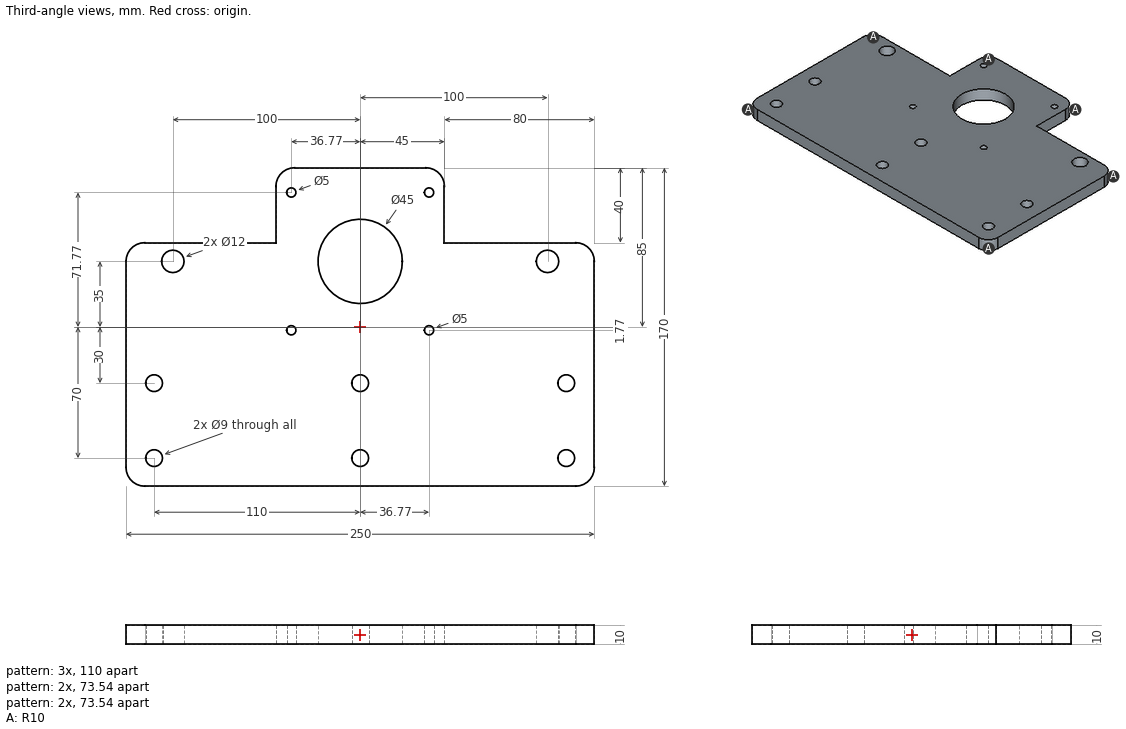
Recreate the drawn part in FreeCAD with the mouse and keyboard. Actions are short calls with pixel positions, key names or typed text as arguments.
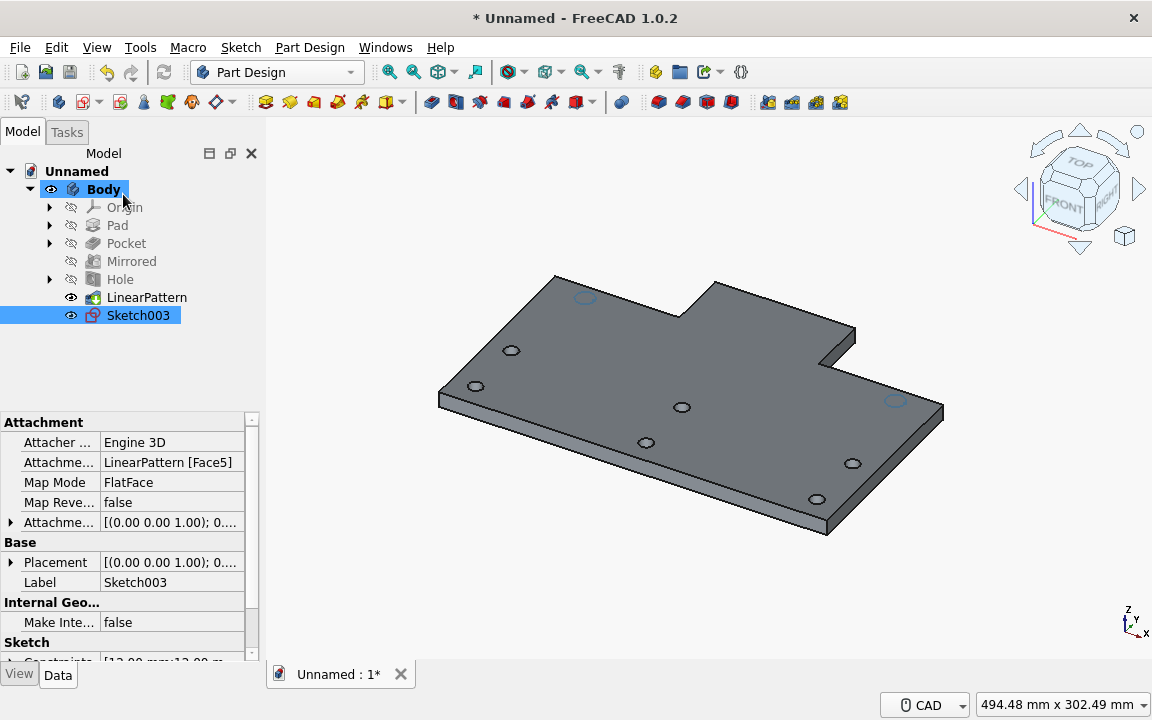
click(432, 102)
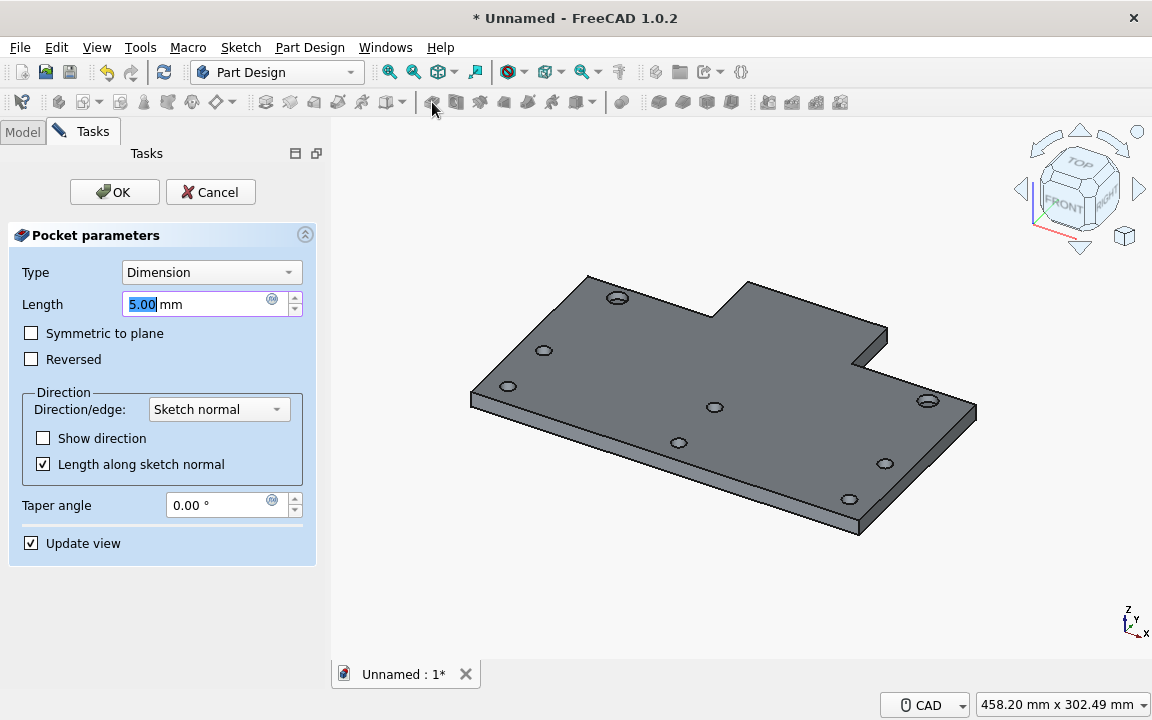
click(212, 272)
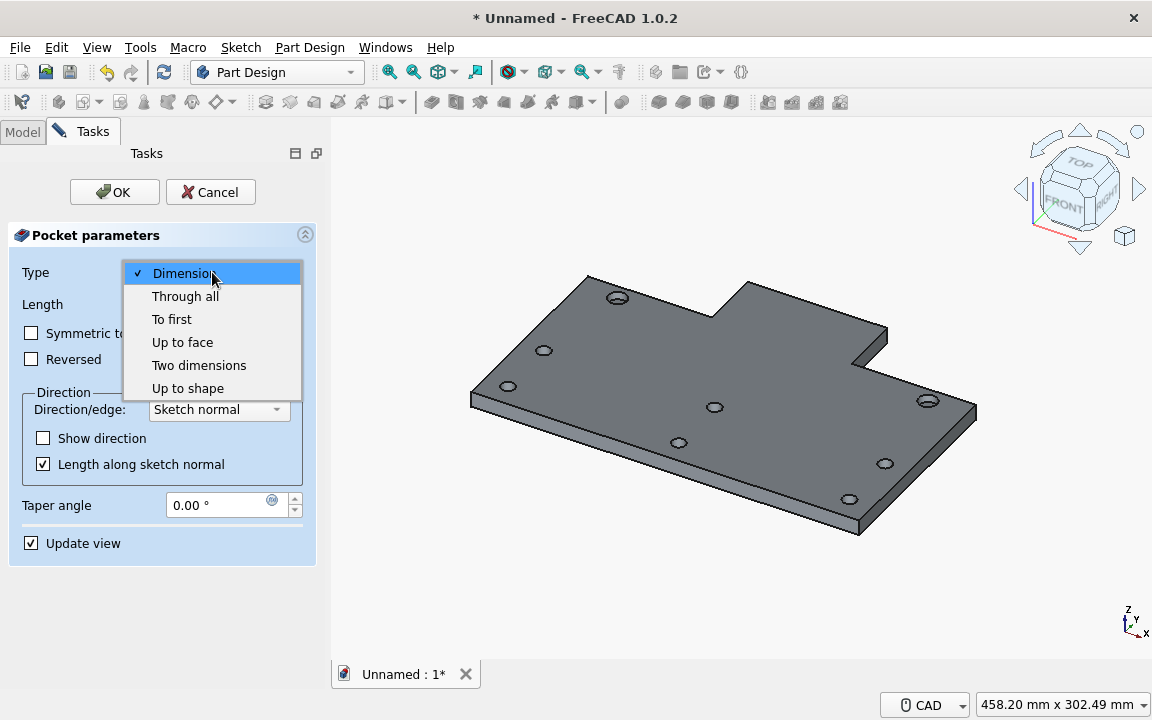
click(212, 296)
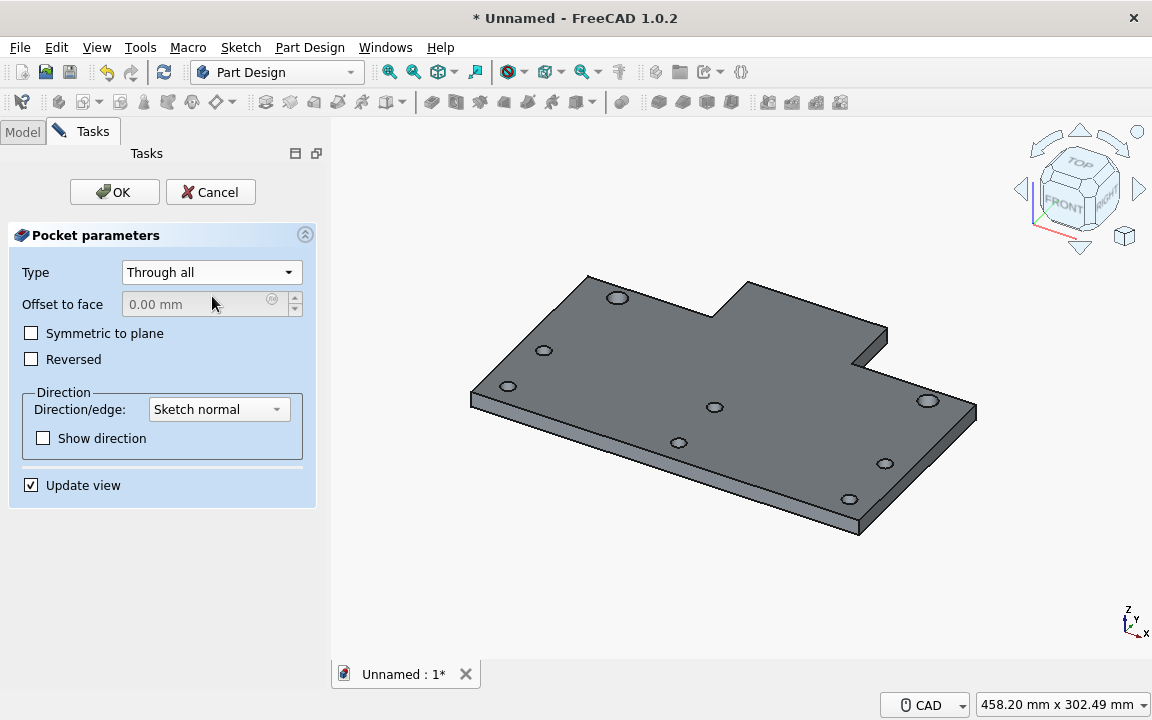
click(115, 192)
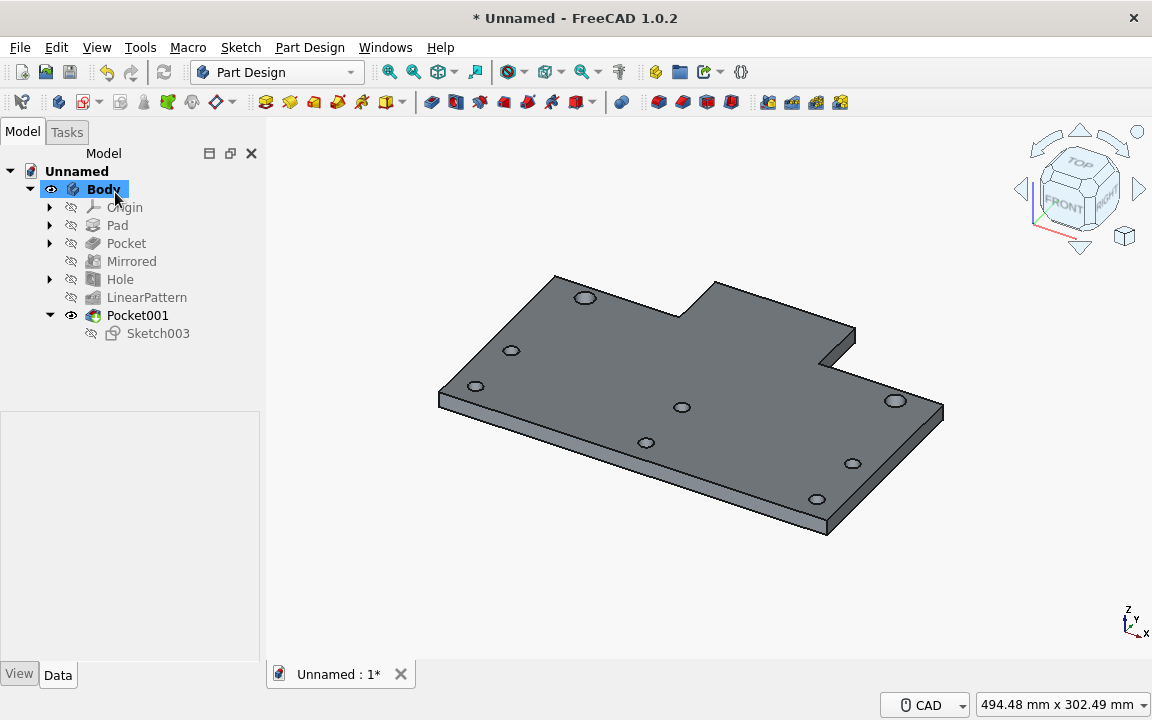
click(731, 358)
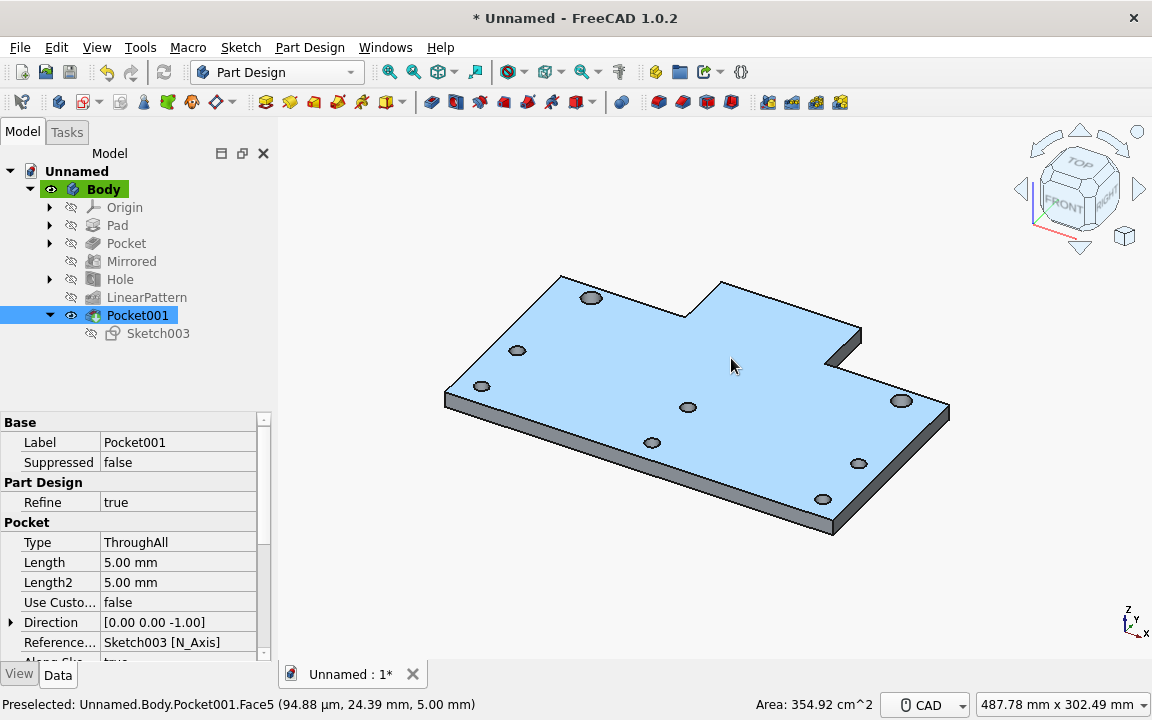
click(84, 102)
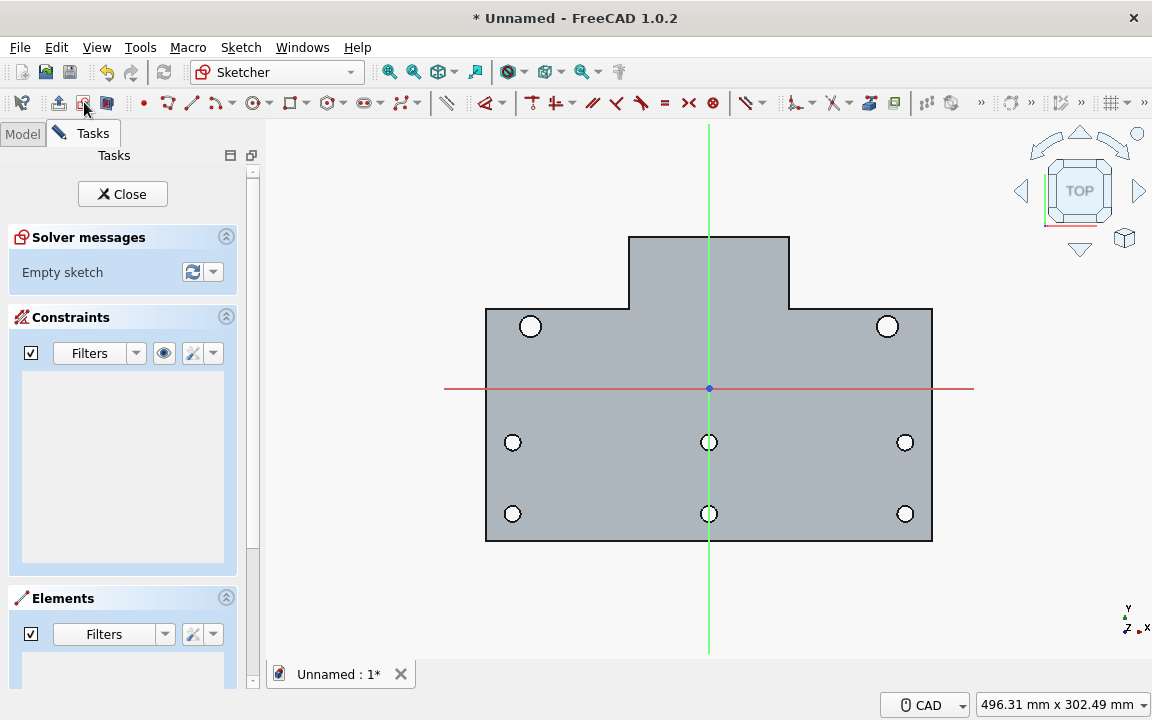
scroll(739, 316, up, 6)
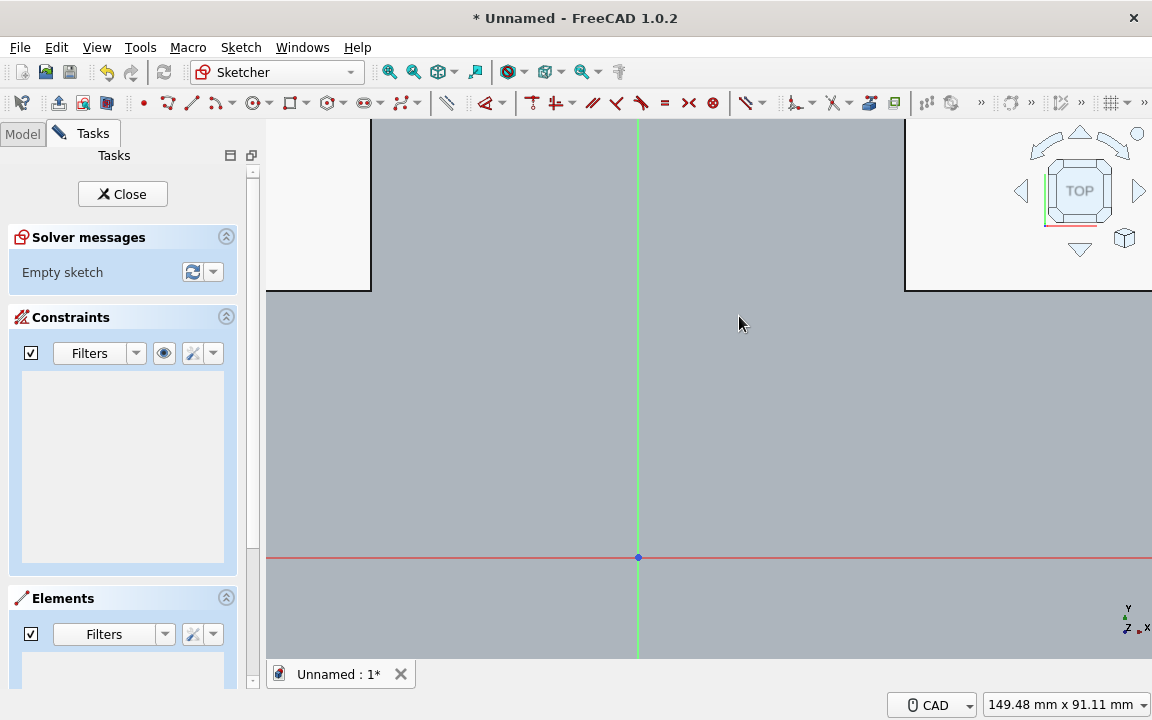
click(254, 104)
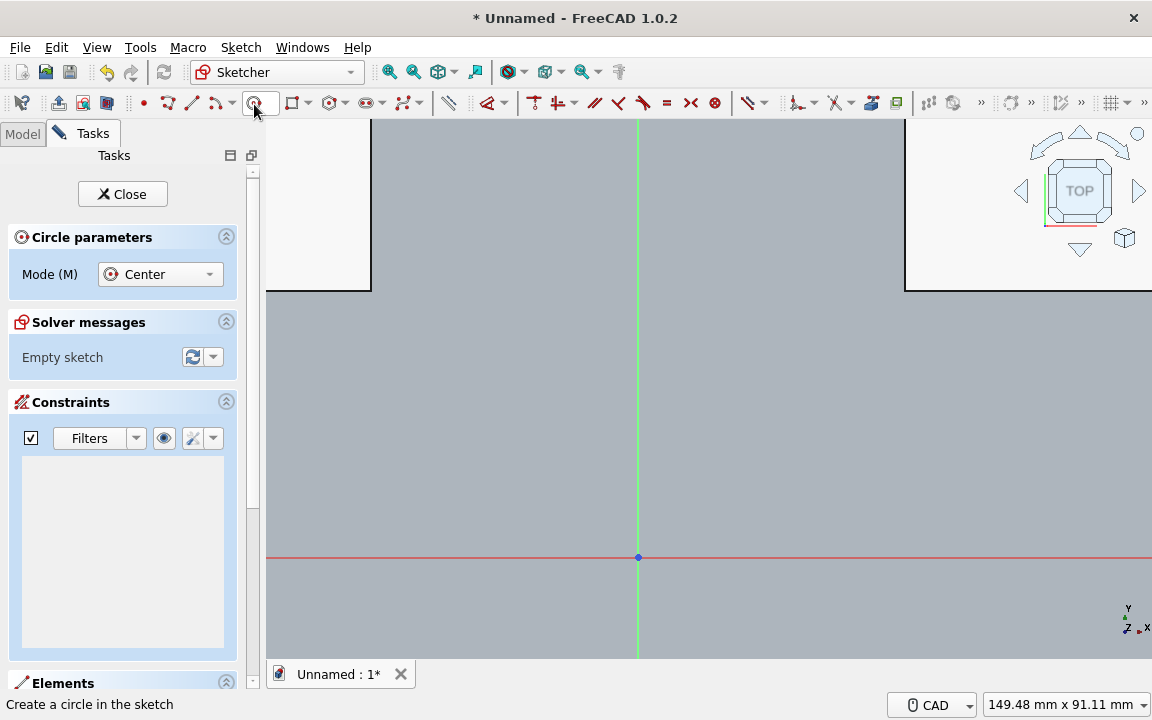
click(638, 350)
move(732, 256)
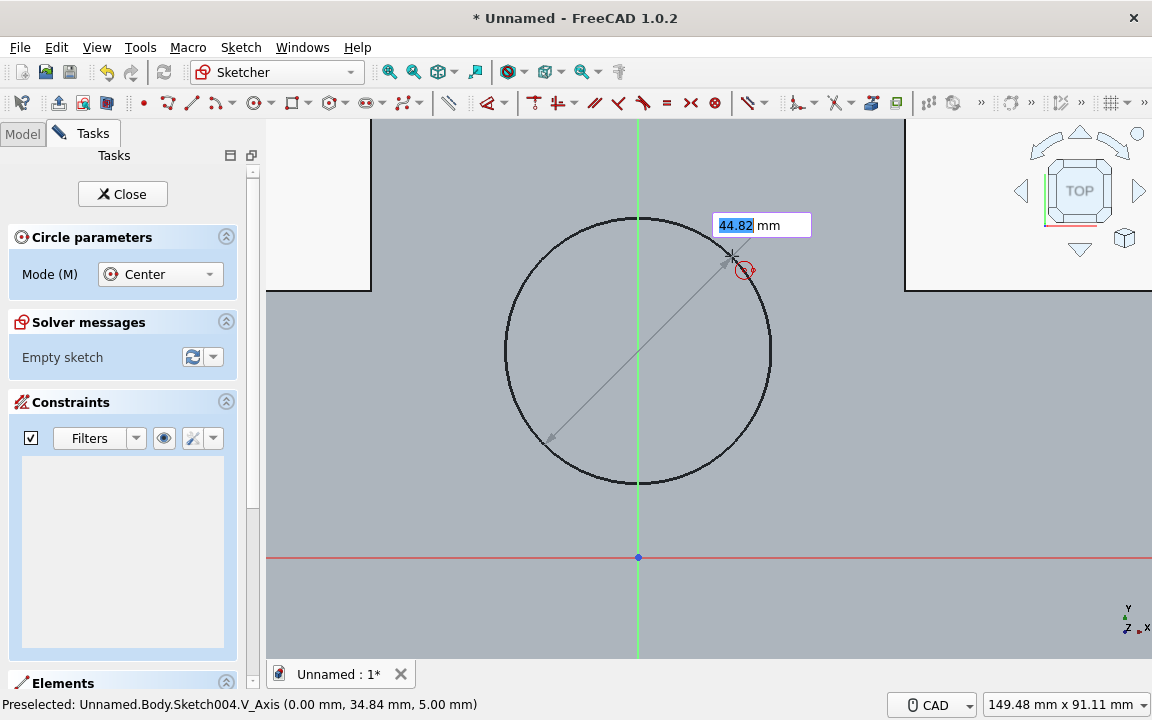
text(45)
key(Return)
key(Escape)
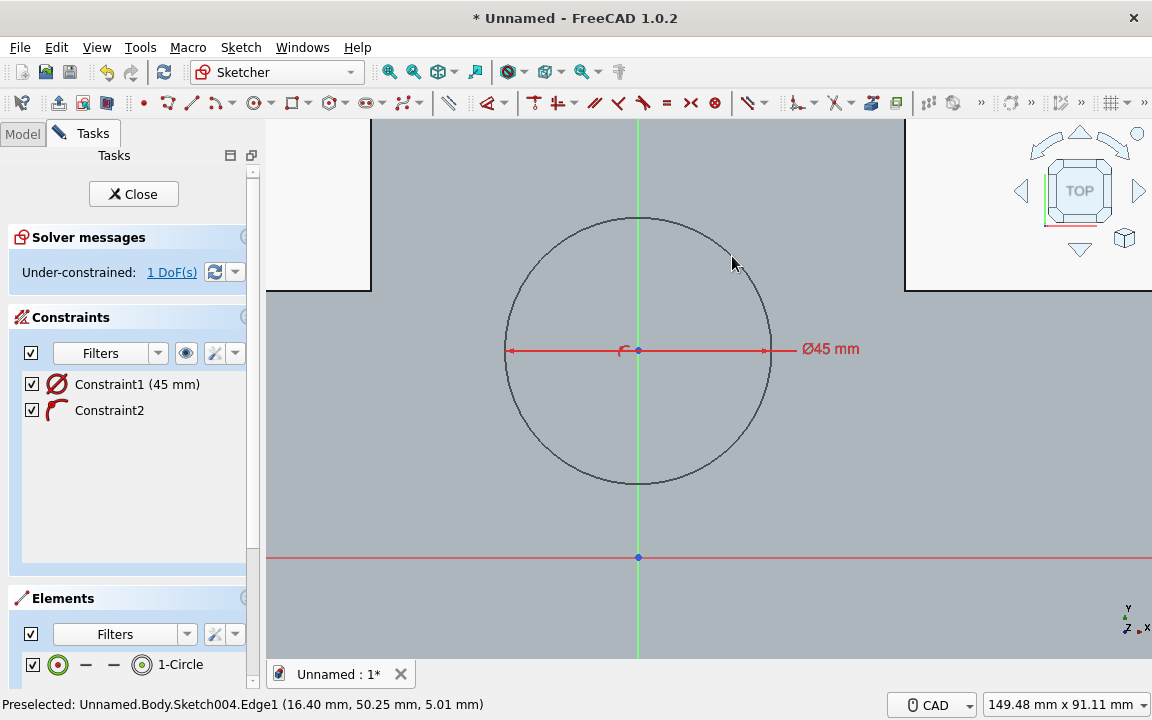
click(488, 104)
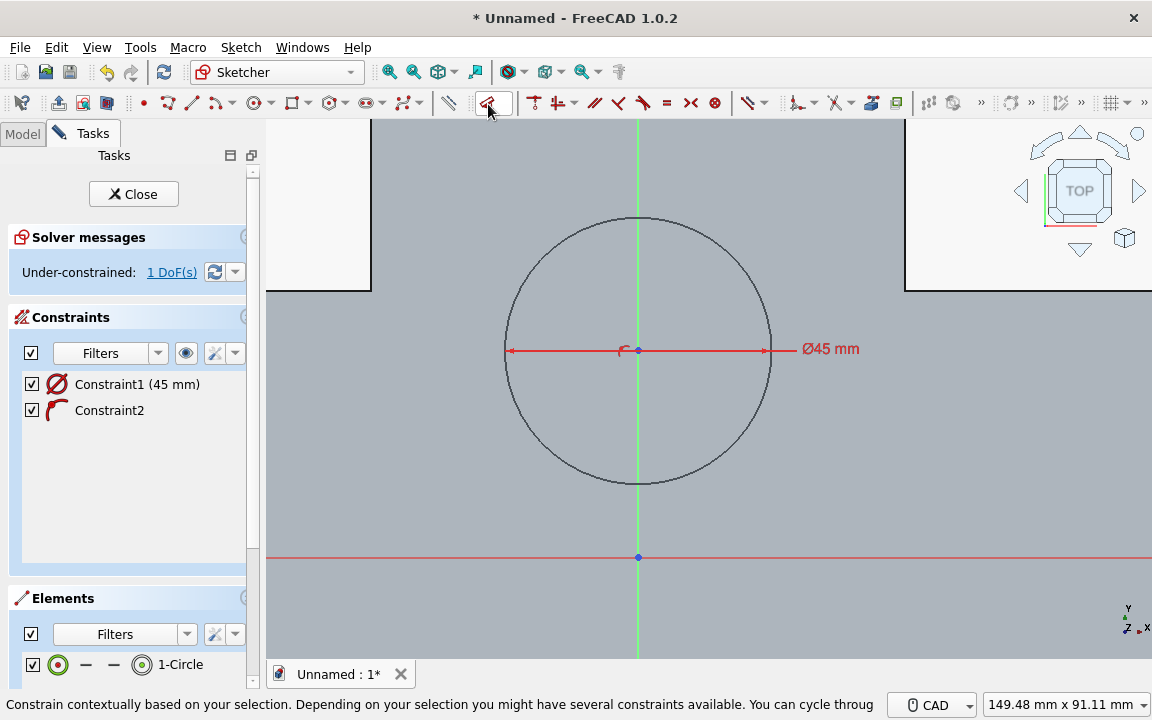
click(638, 351)
click(672, 454)